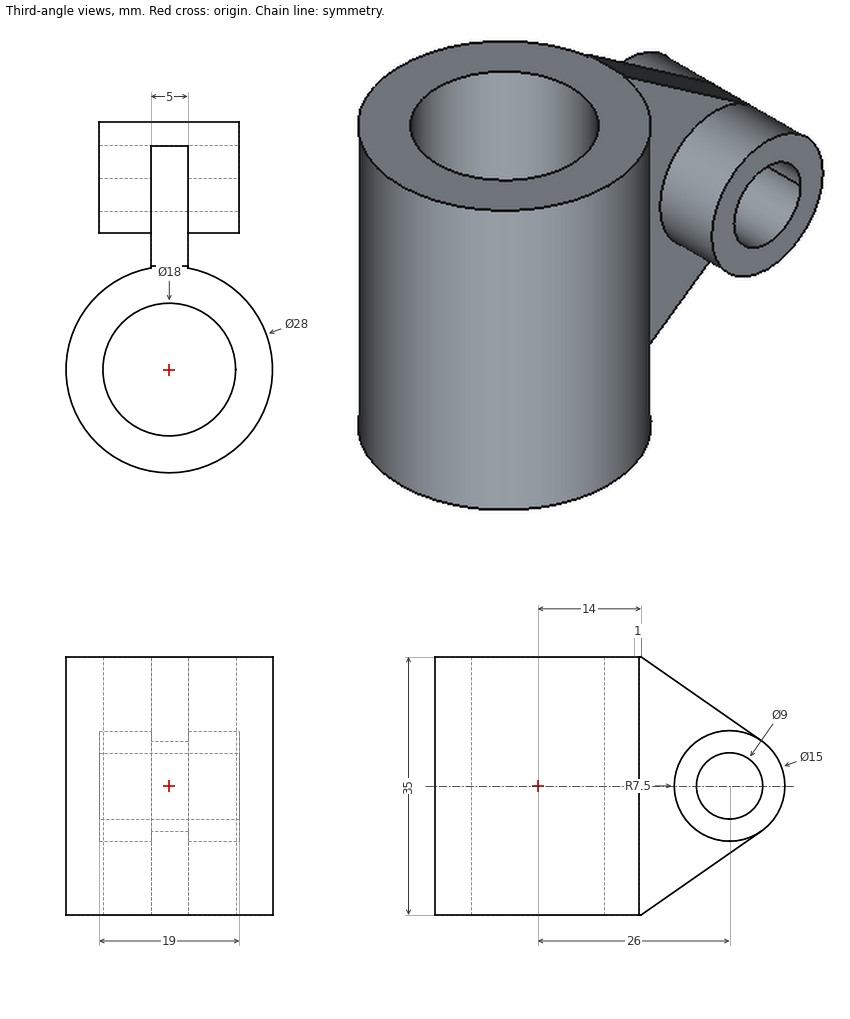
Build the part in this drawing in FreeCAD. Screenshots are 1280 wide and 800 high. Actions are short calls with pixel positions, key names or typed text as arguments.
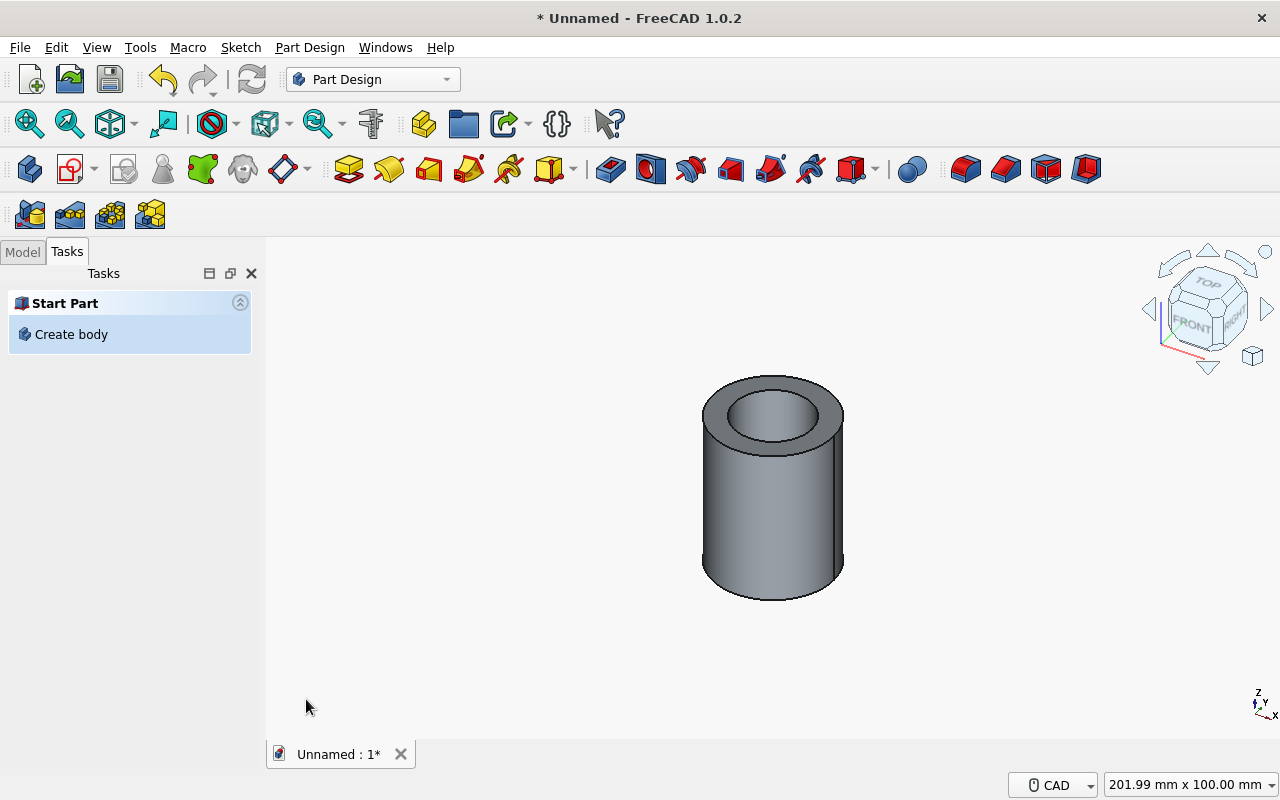
click(70, 170)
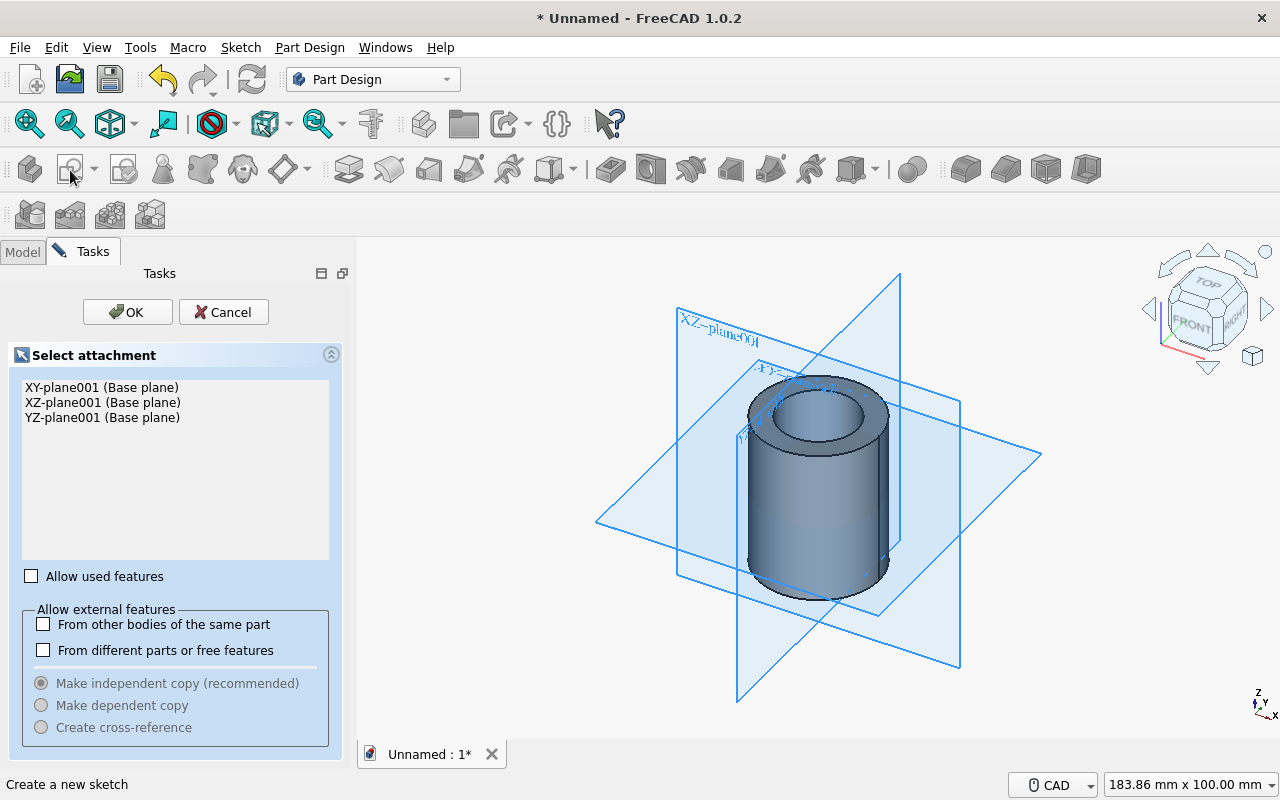
click(82, 418)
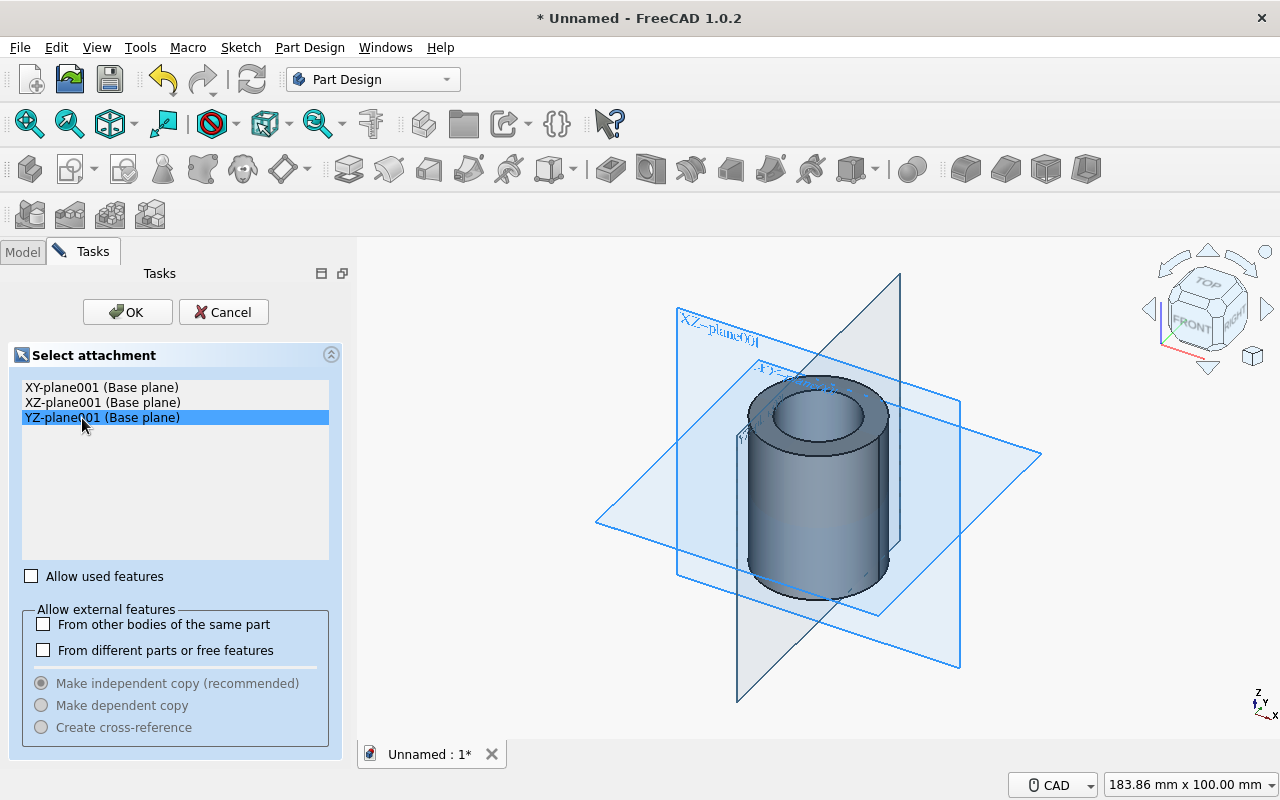
click(128, 312)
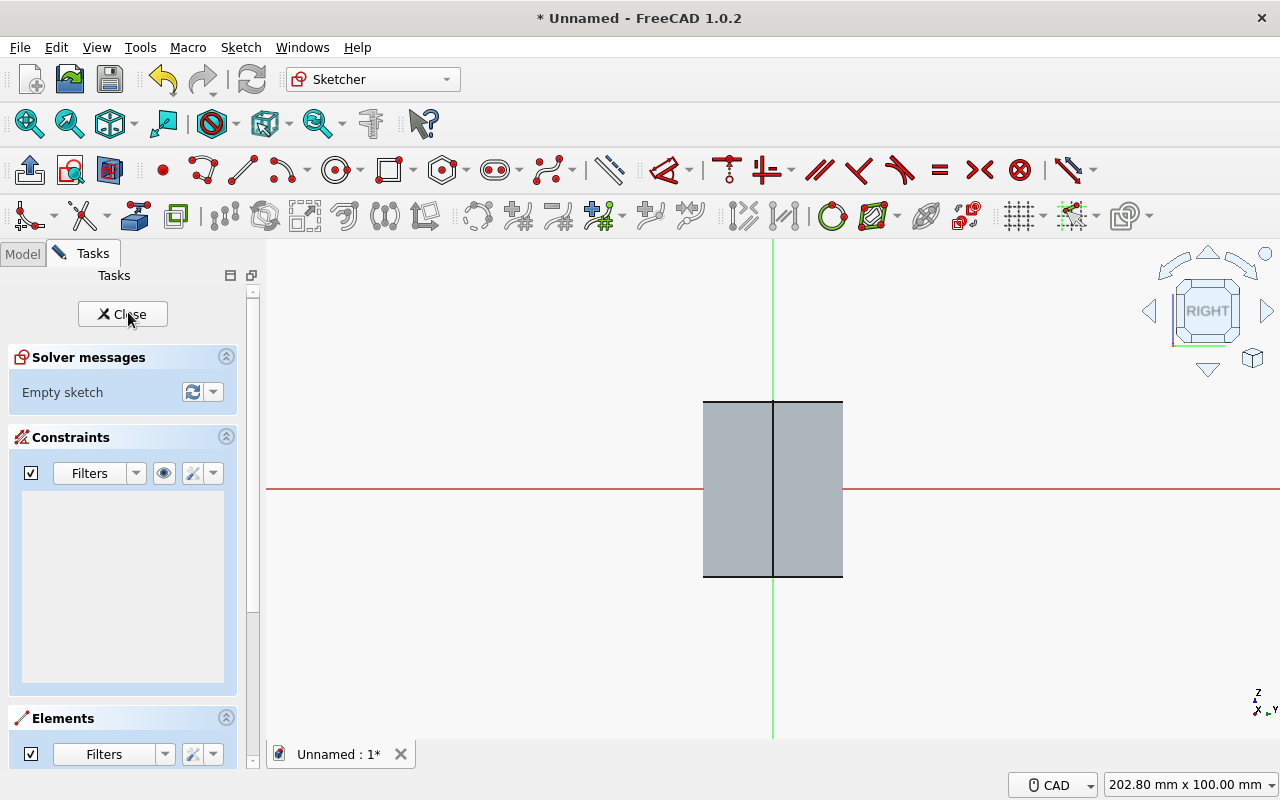
scroll(922, 489, up, 6)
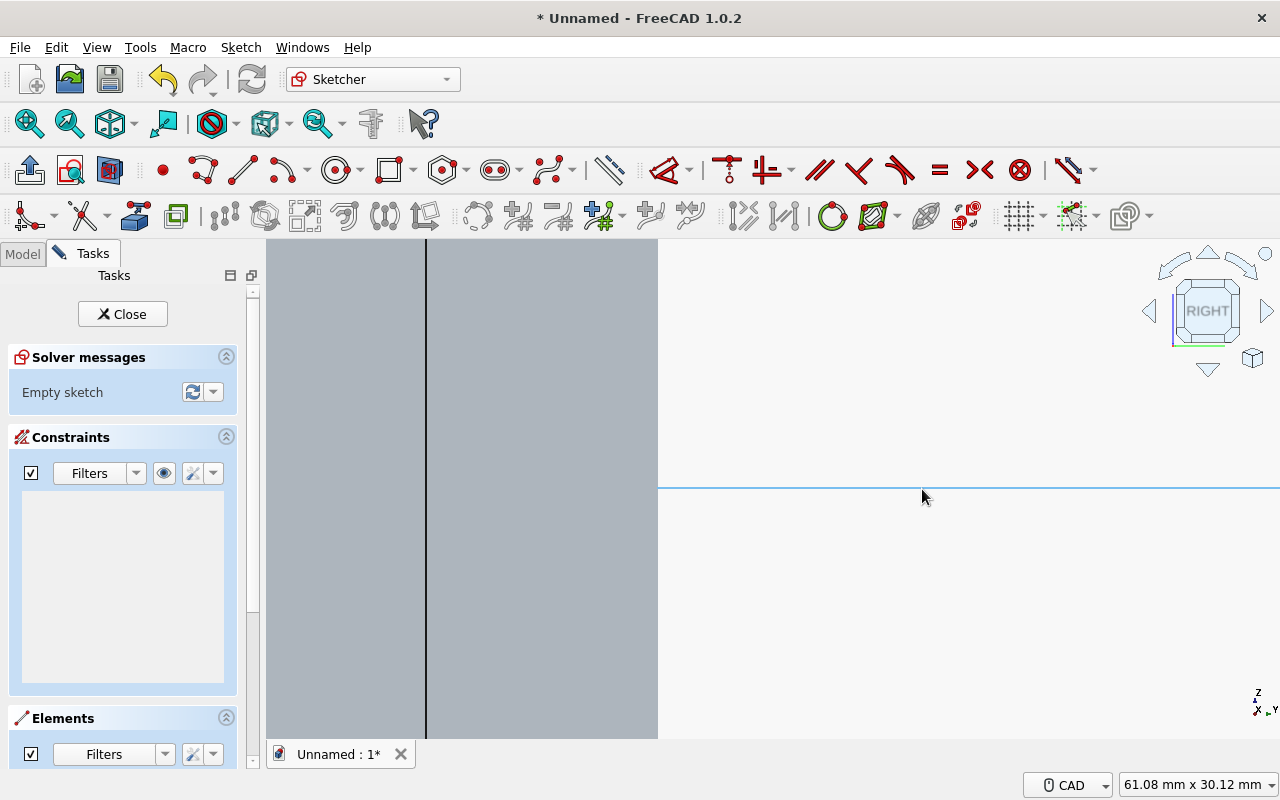
key(g)
key(c)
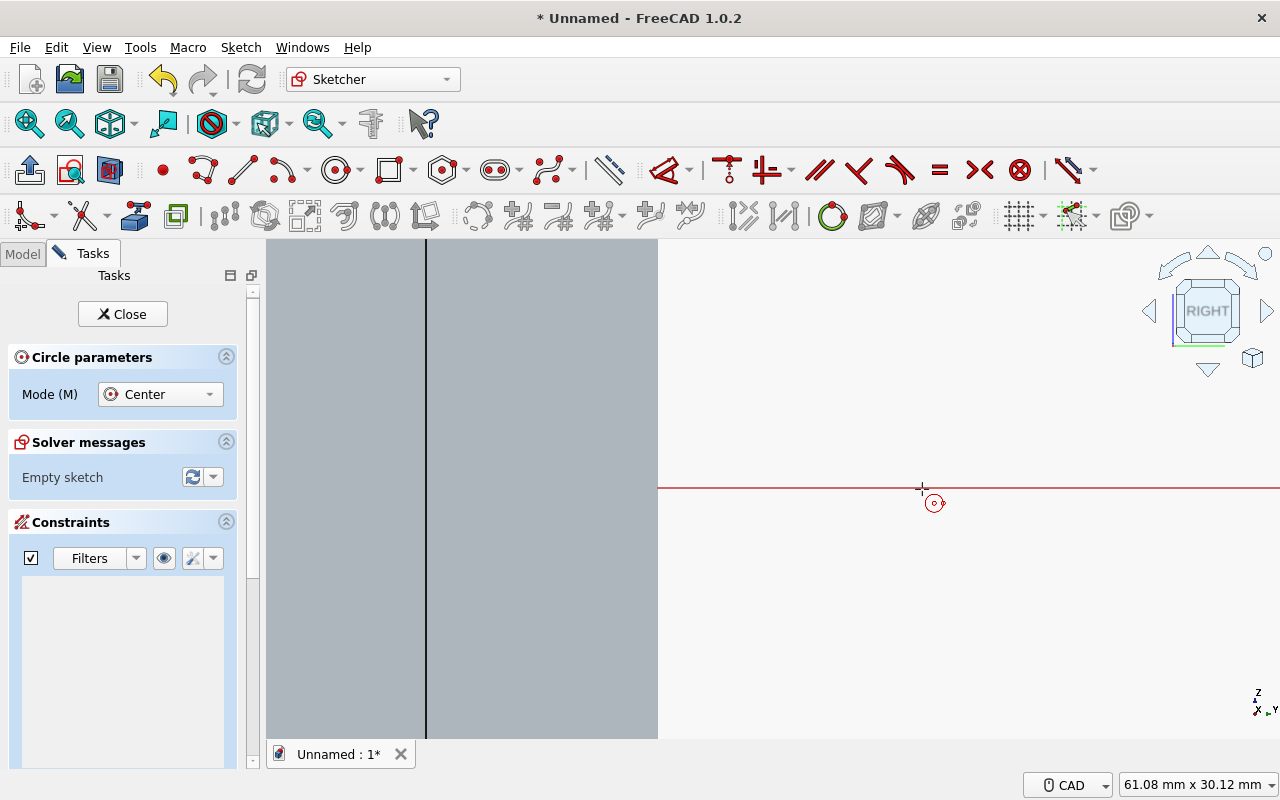
click(857, 488)
click(945, 400)
key(Escape)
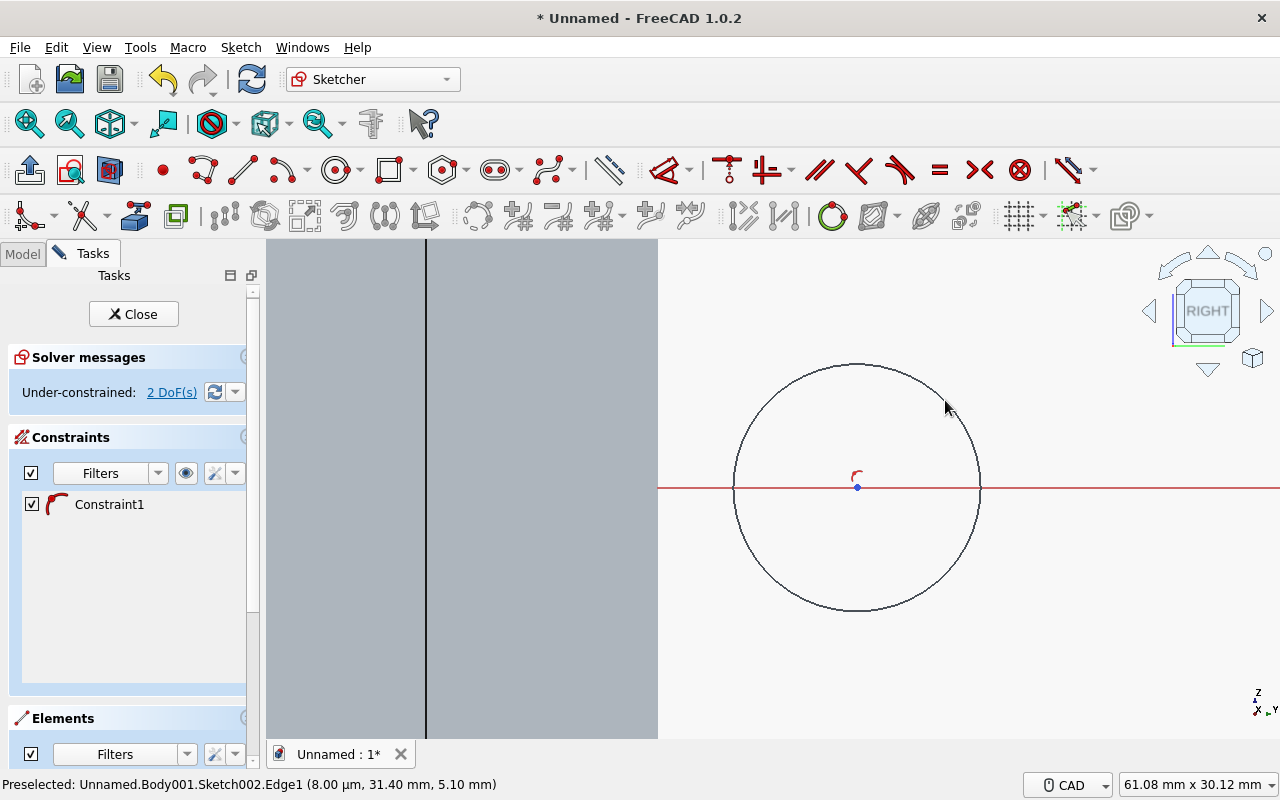
click(664, 170)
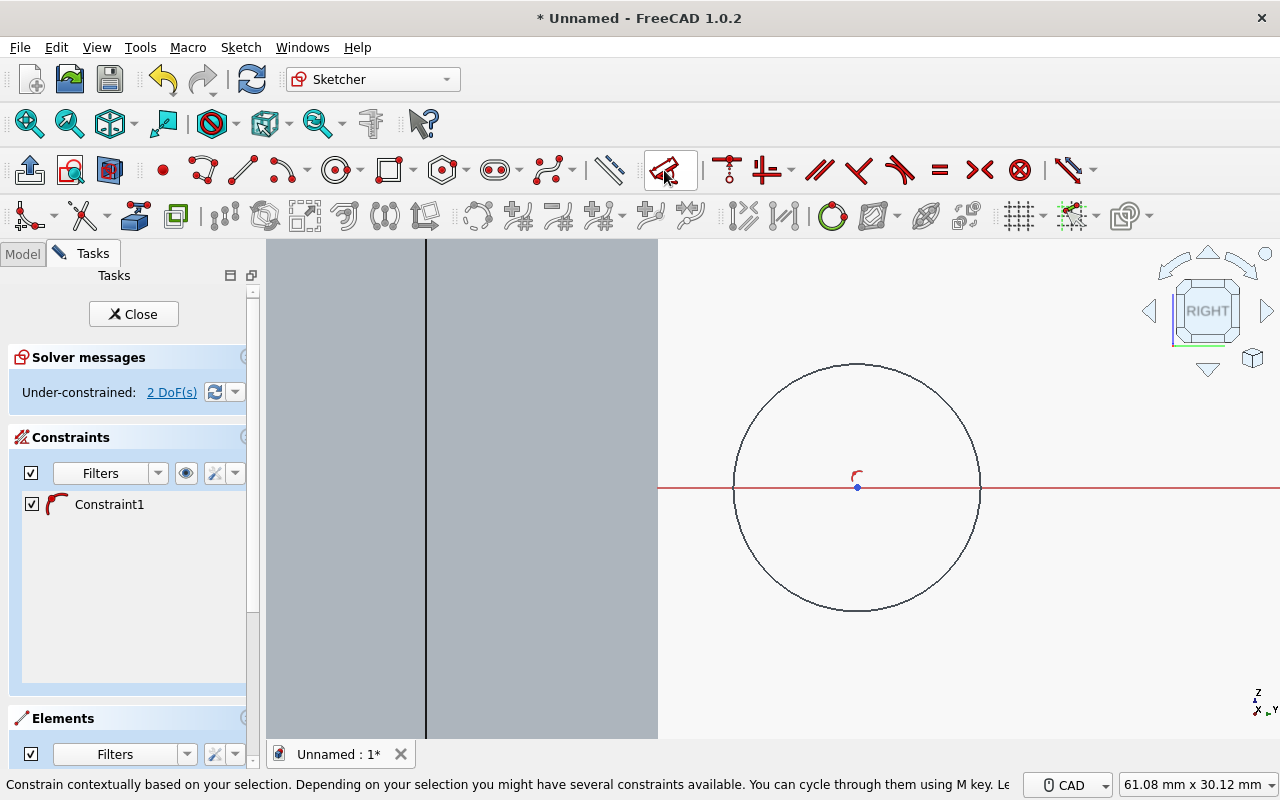
click(944, 400)
click(967, 377)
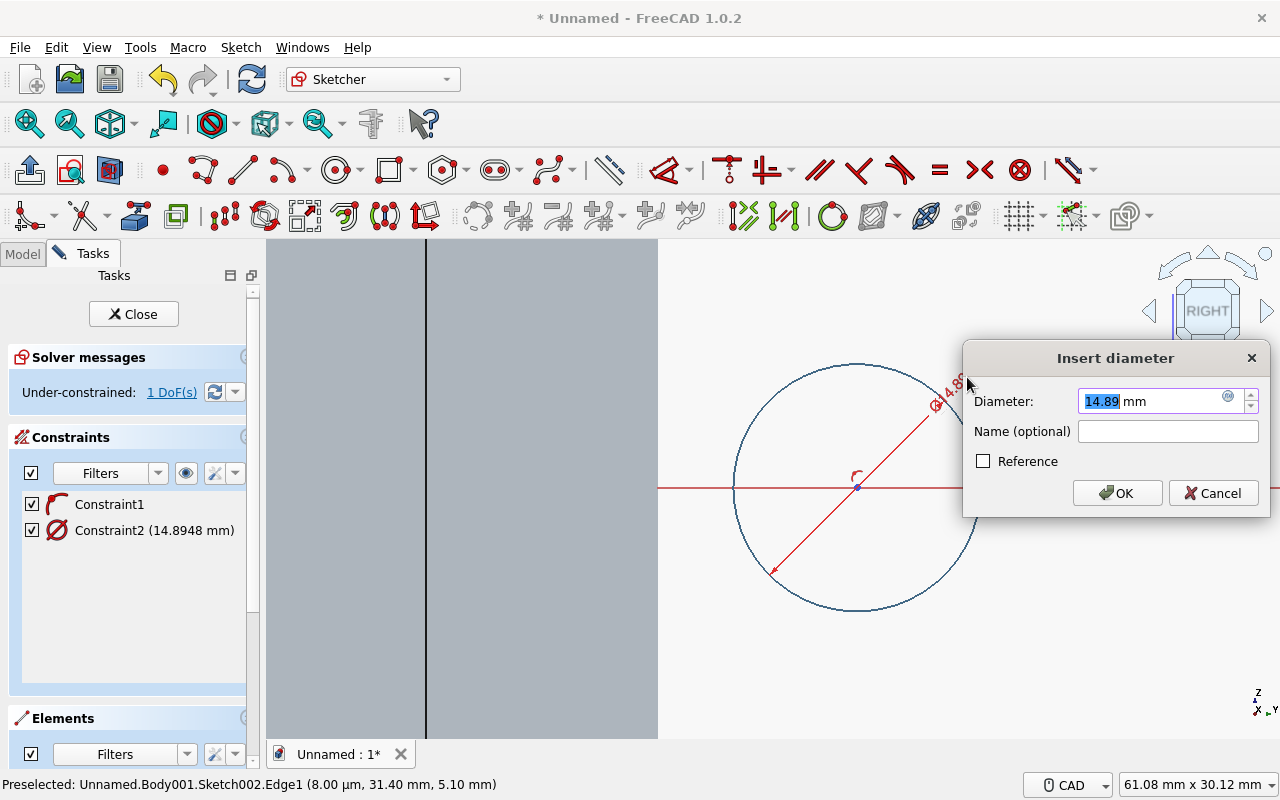
text(15)
key(Return)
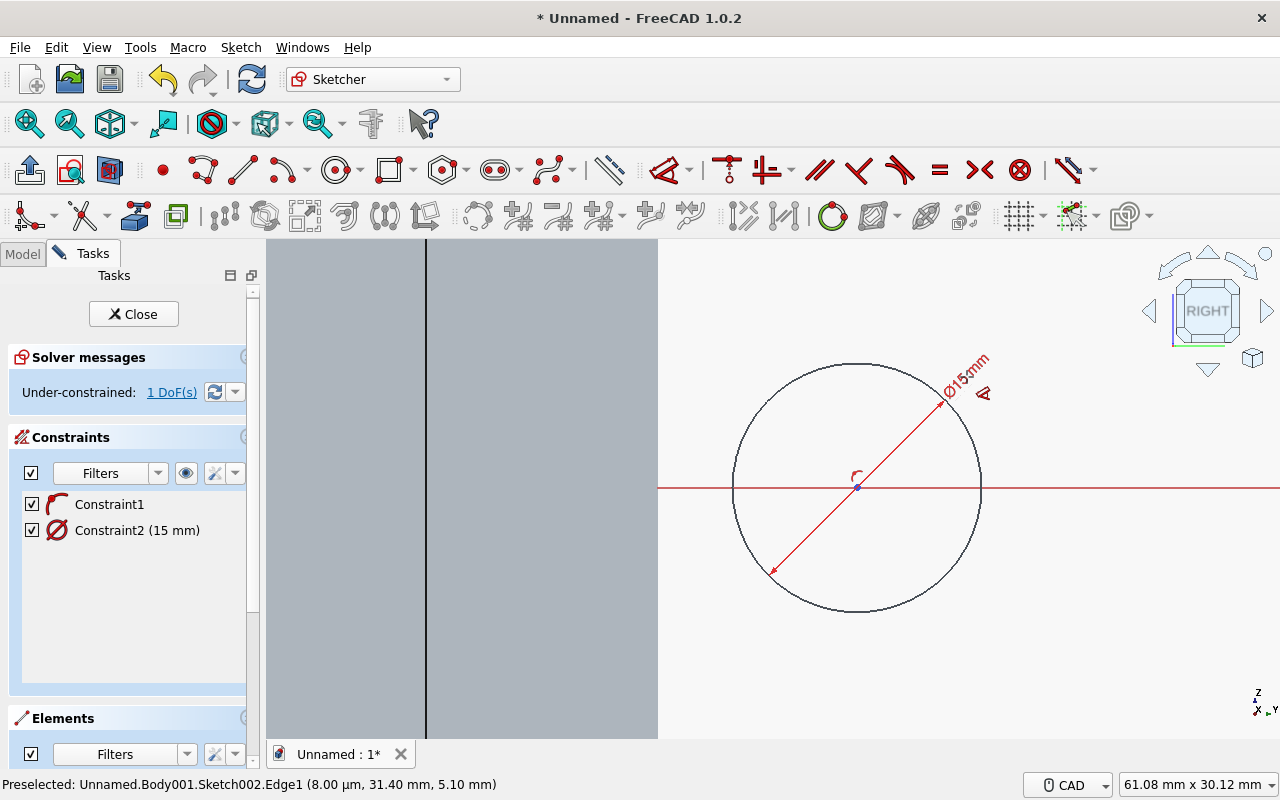
click(857, 488)
click(641, 522)